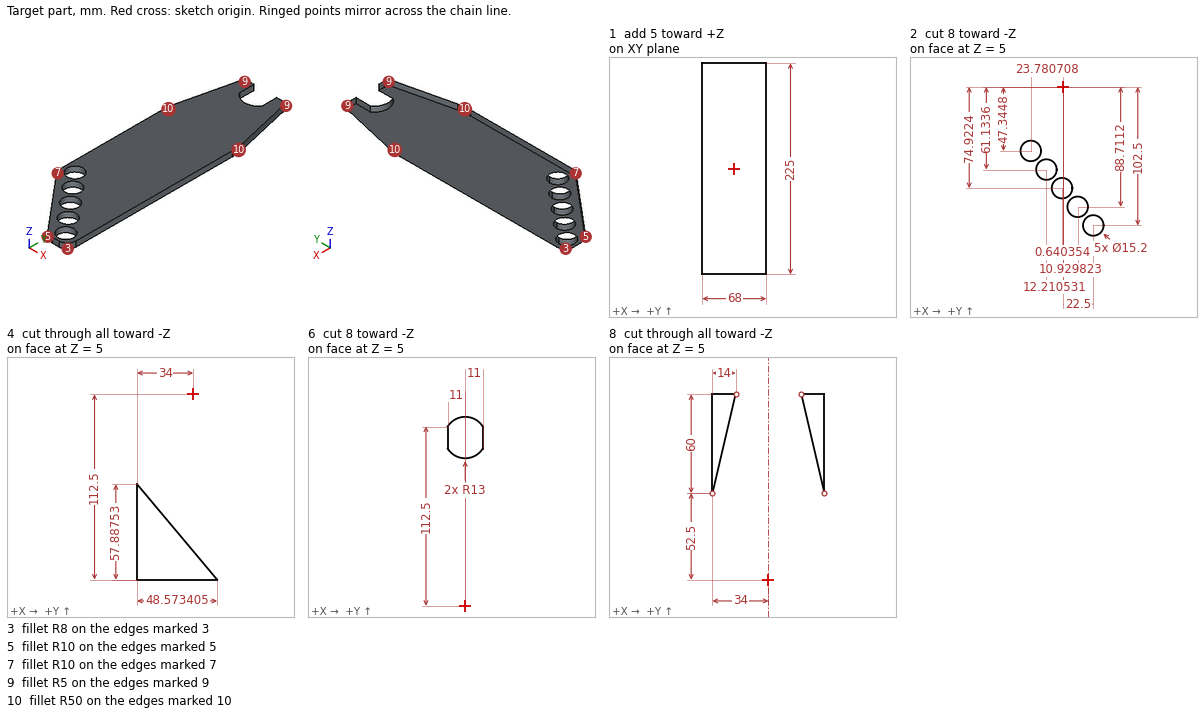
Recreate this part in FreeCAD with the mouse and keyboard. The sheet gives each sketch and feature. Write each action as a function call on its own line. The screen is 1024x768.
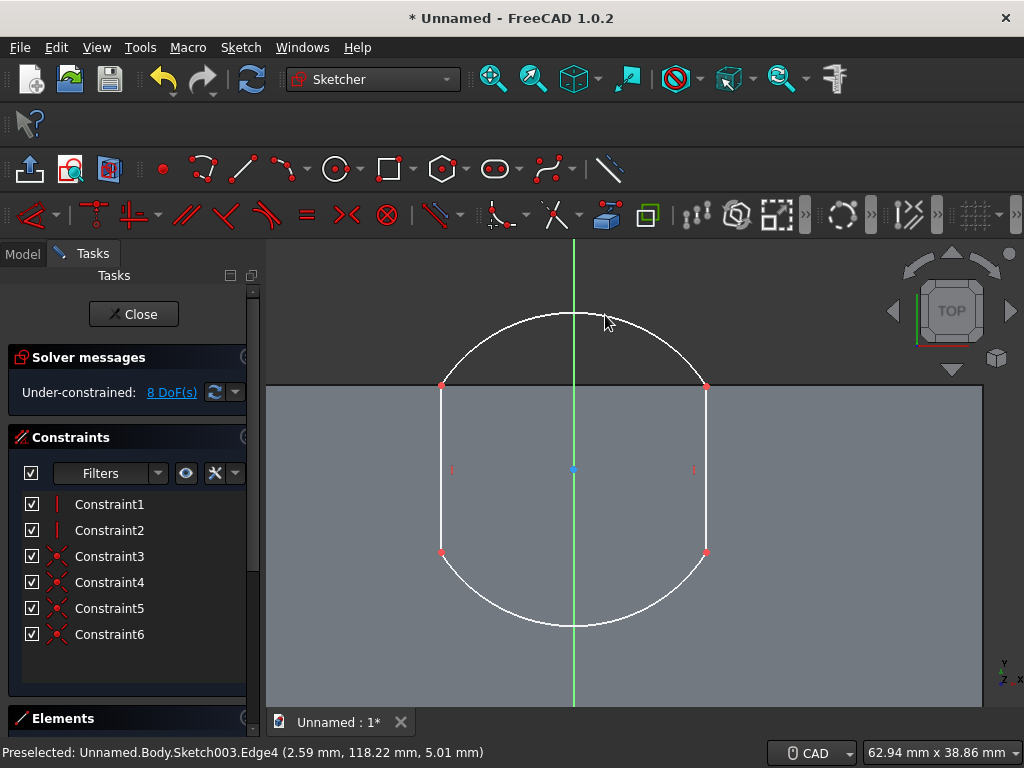
click(512, 614)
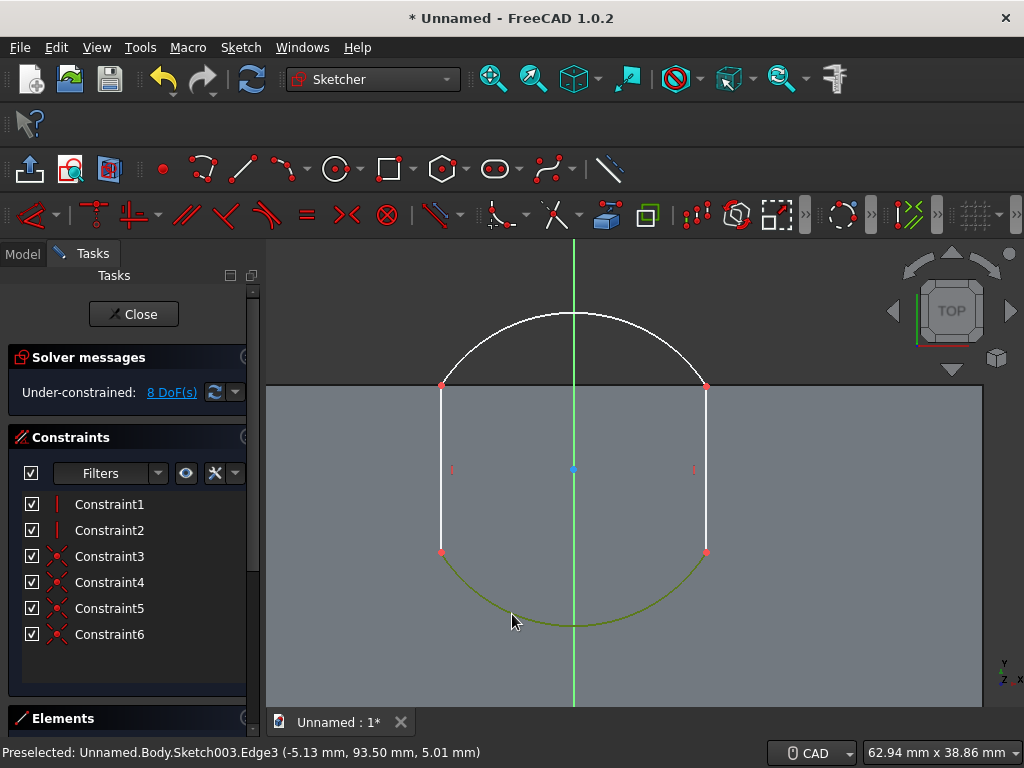
click(635, 325)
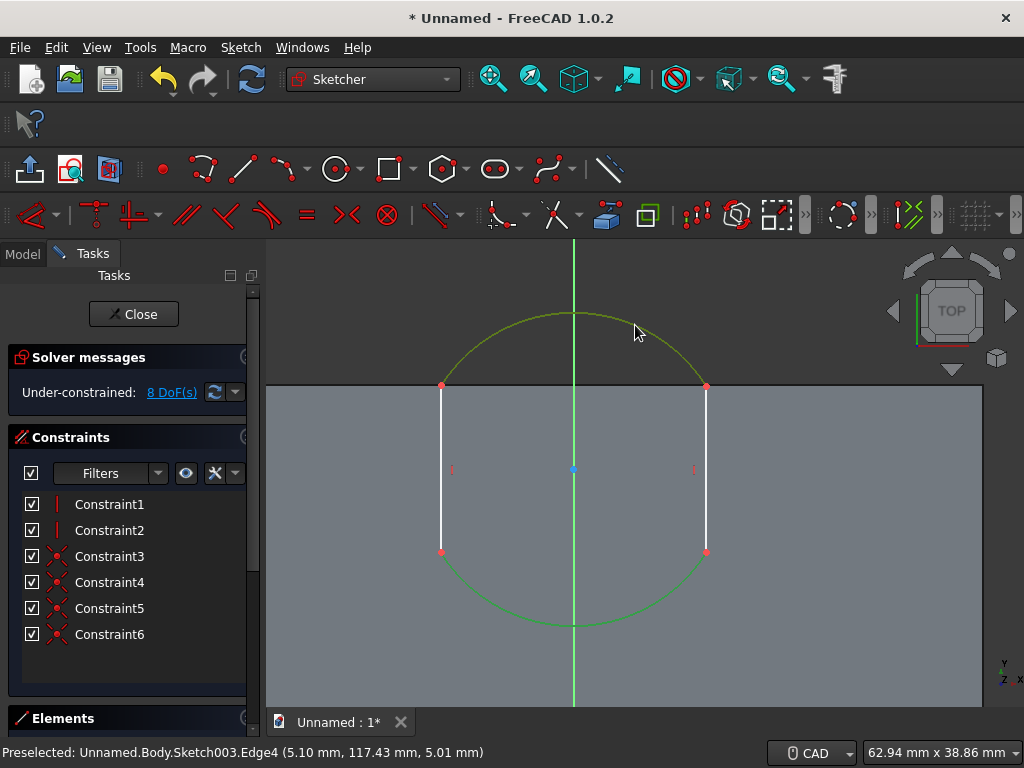
key(c)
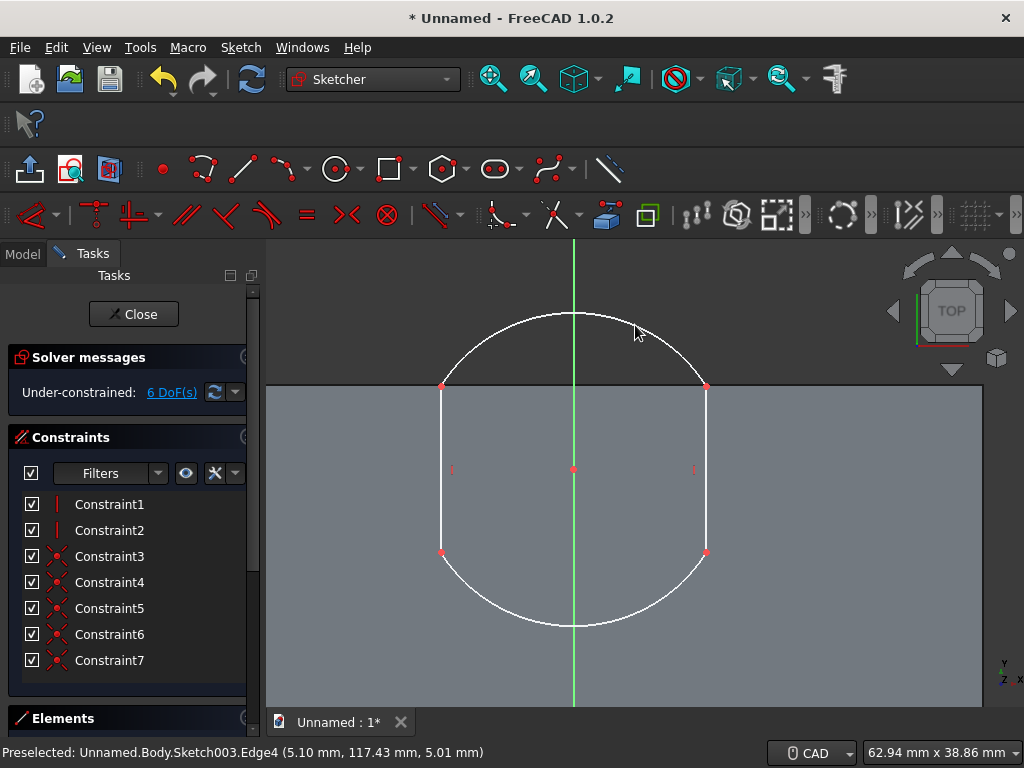
click(512, 614)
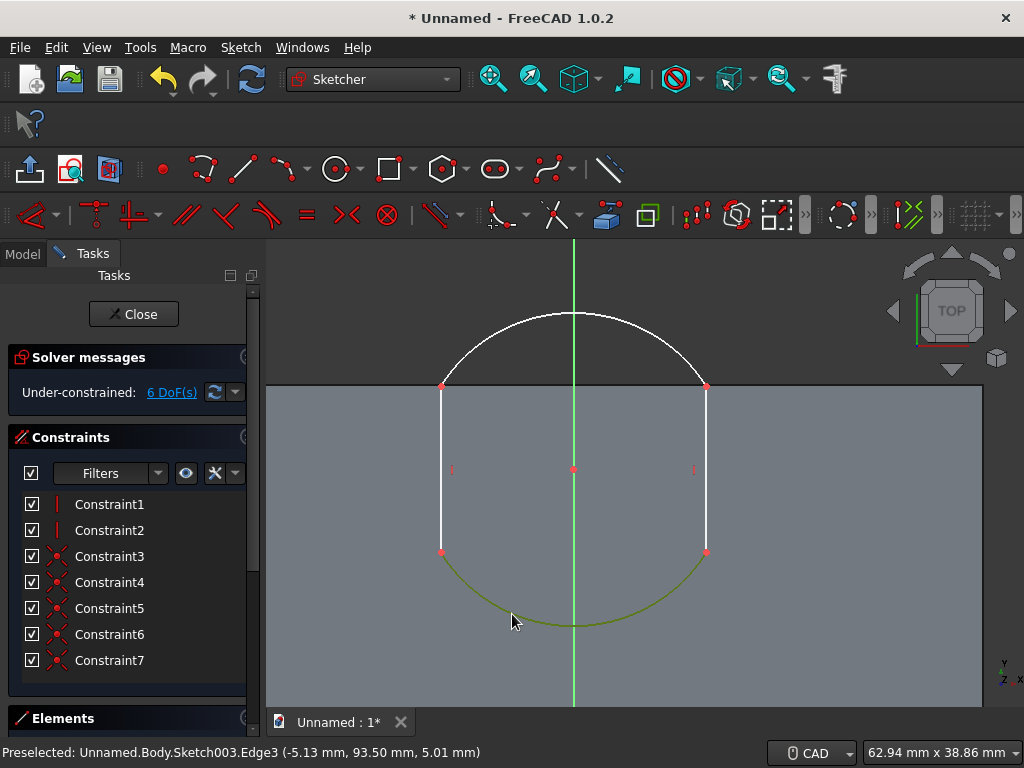
click(635, 326)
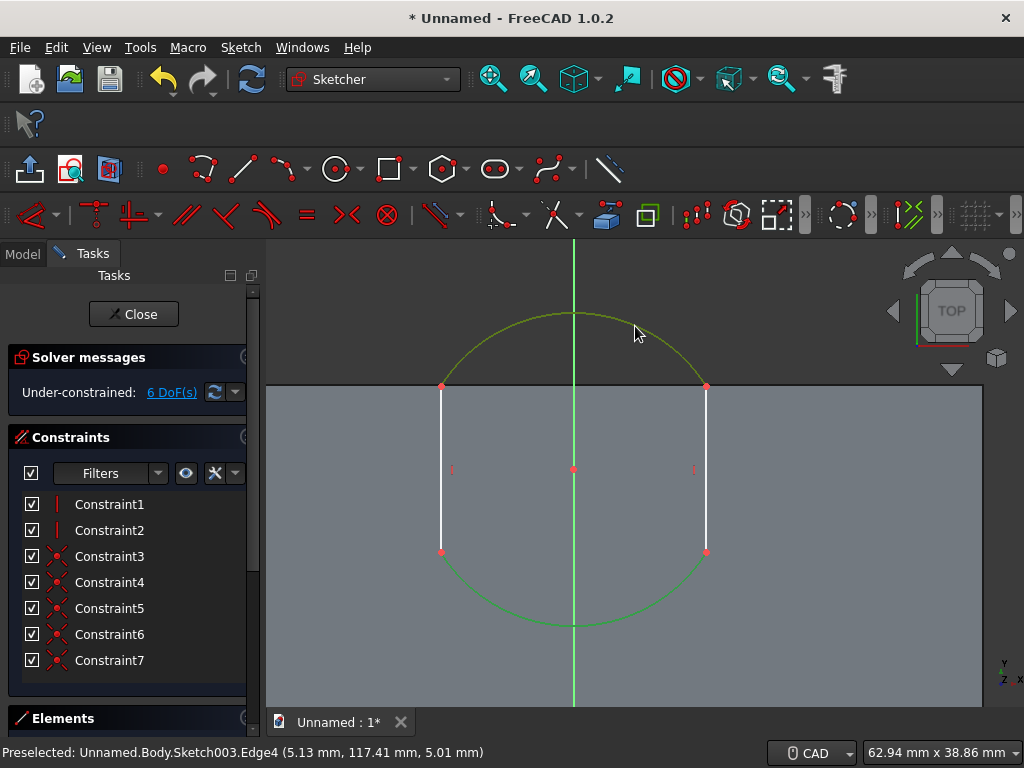
key(e)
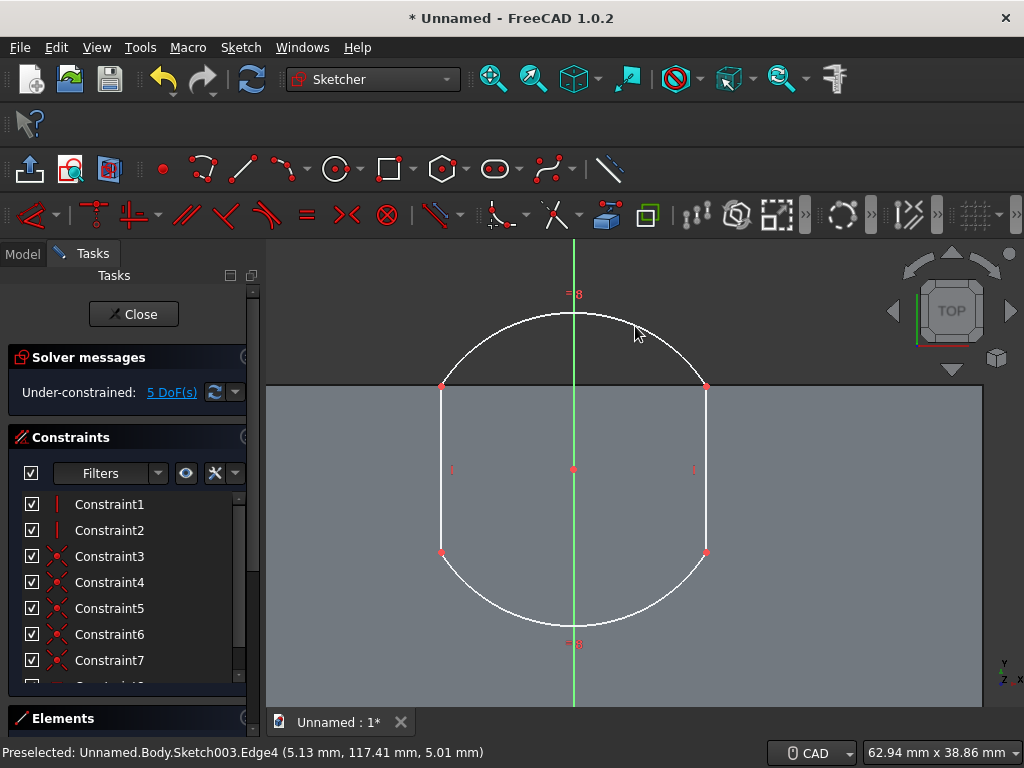
click(574, 470)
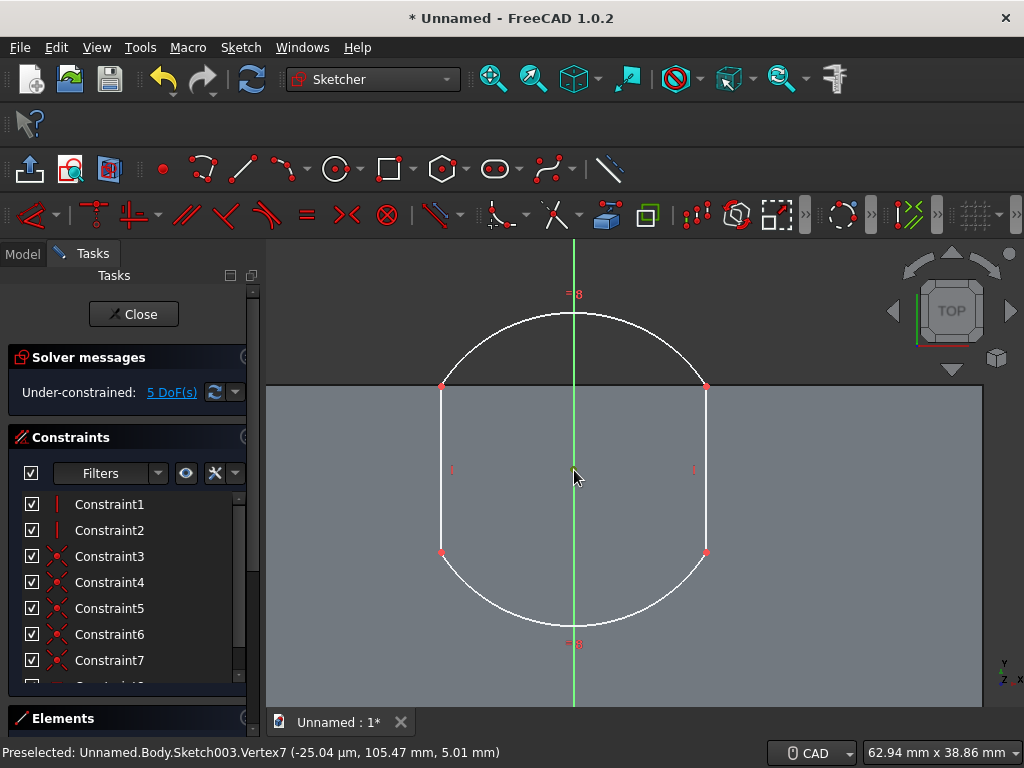
click(574, 591)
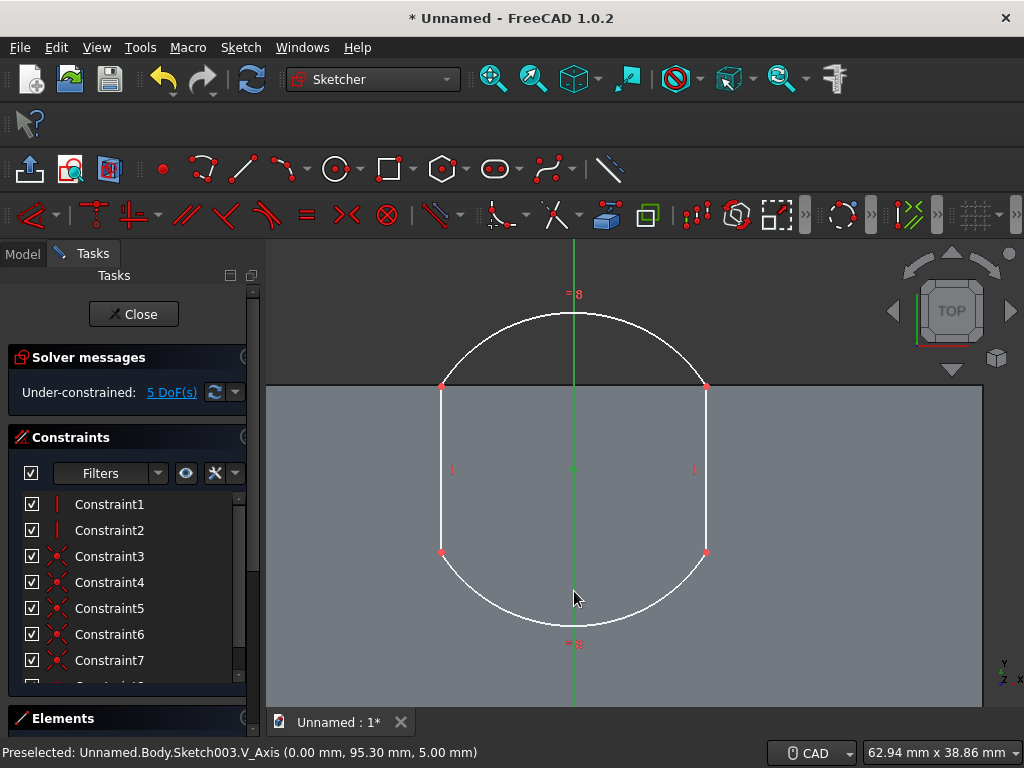
click(94, 216)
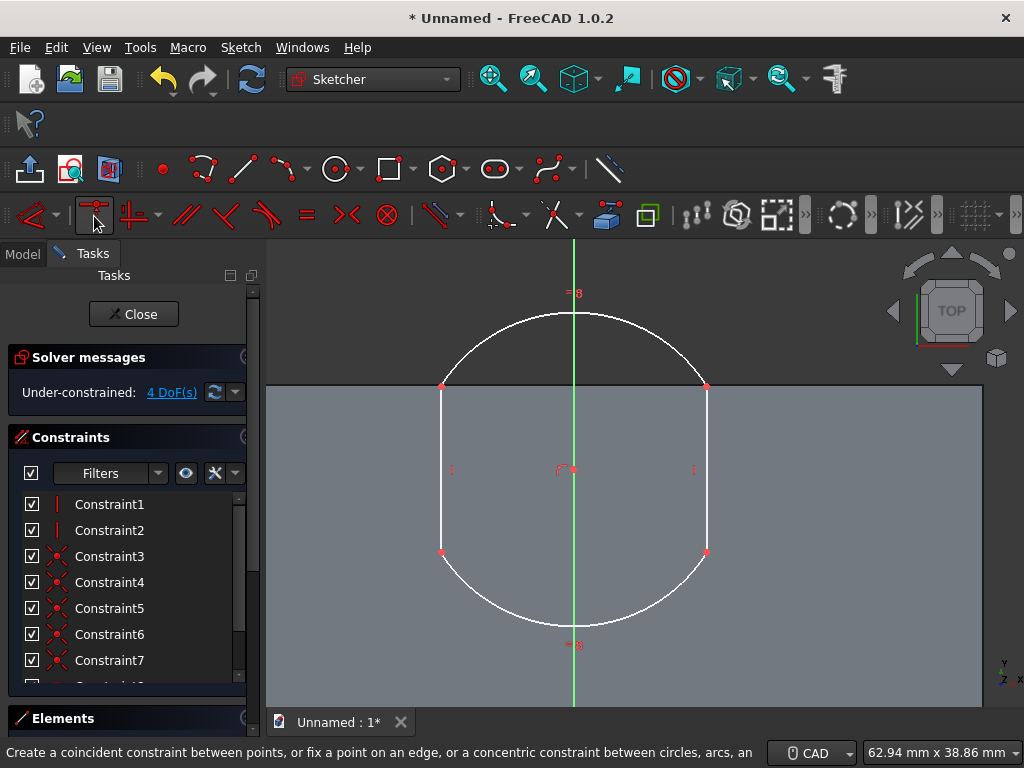
key(d)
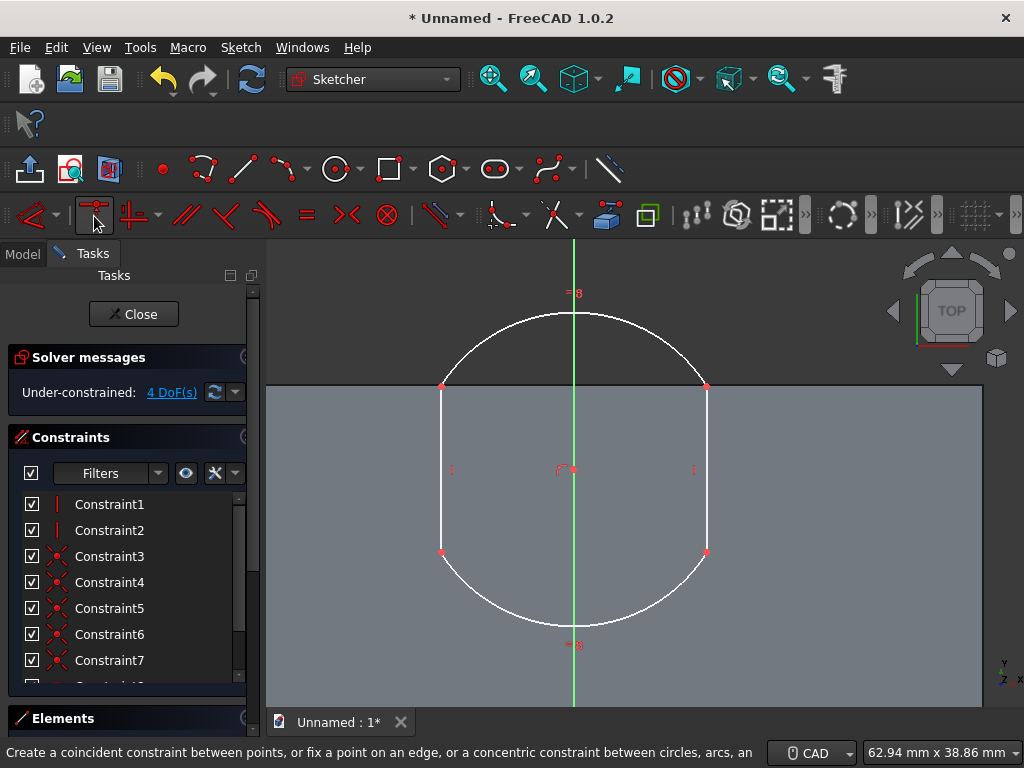
click(512, 614)
click(499, 643)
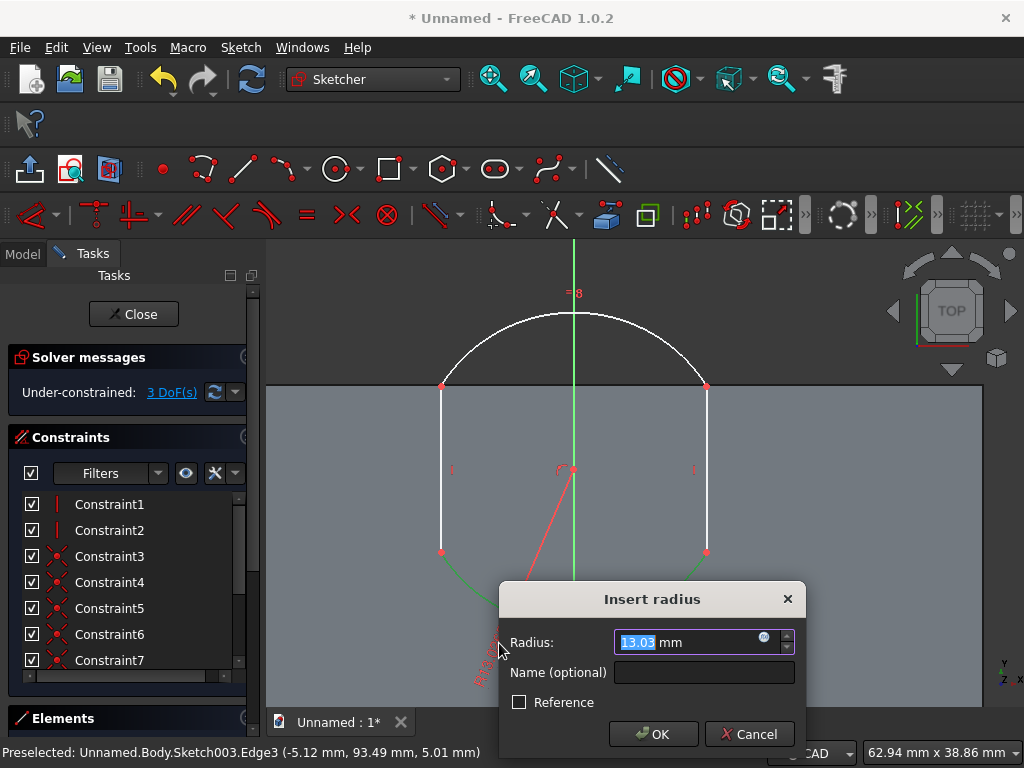
text(13)
key(Return)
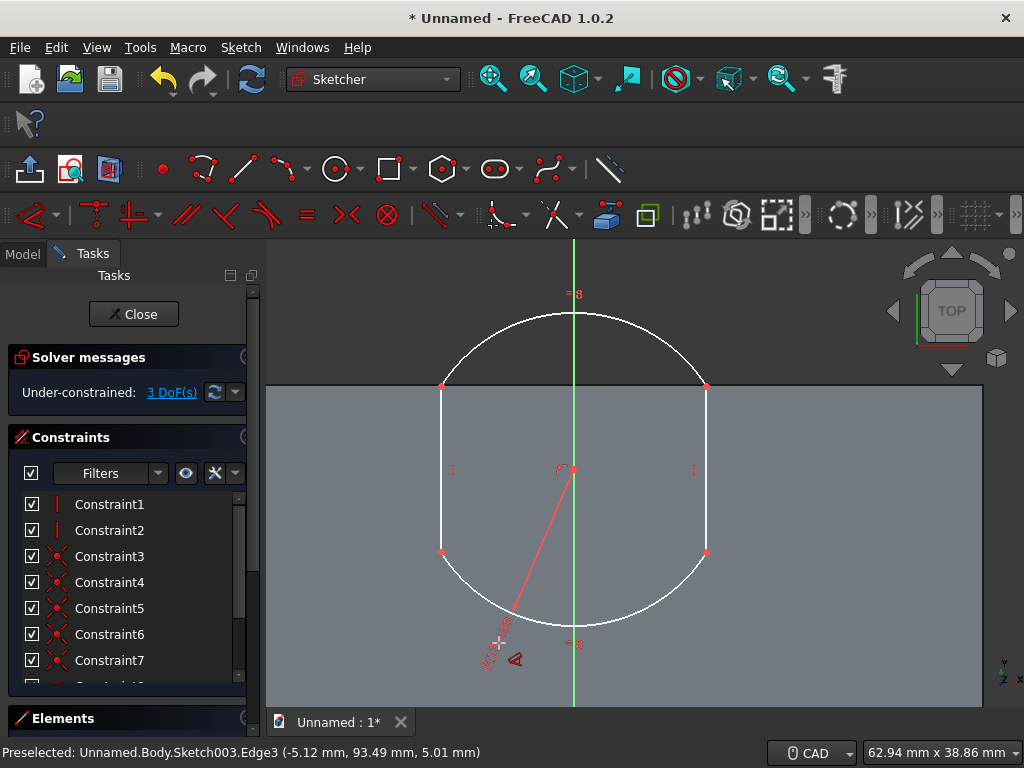
click(441, 386)
click(508, 352)